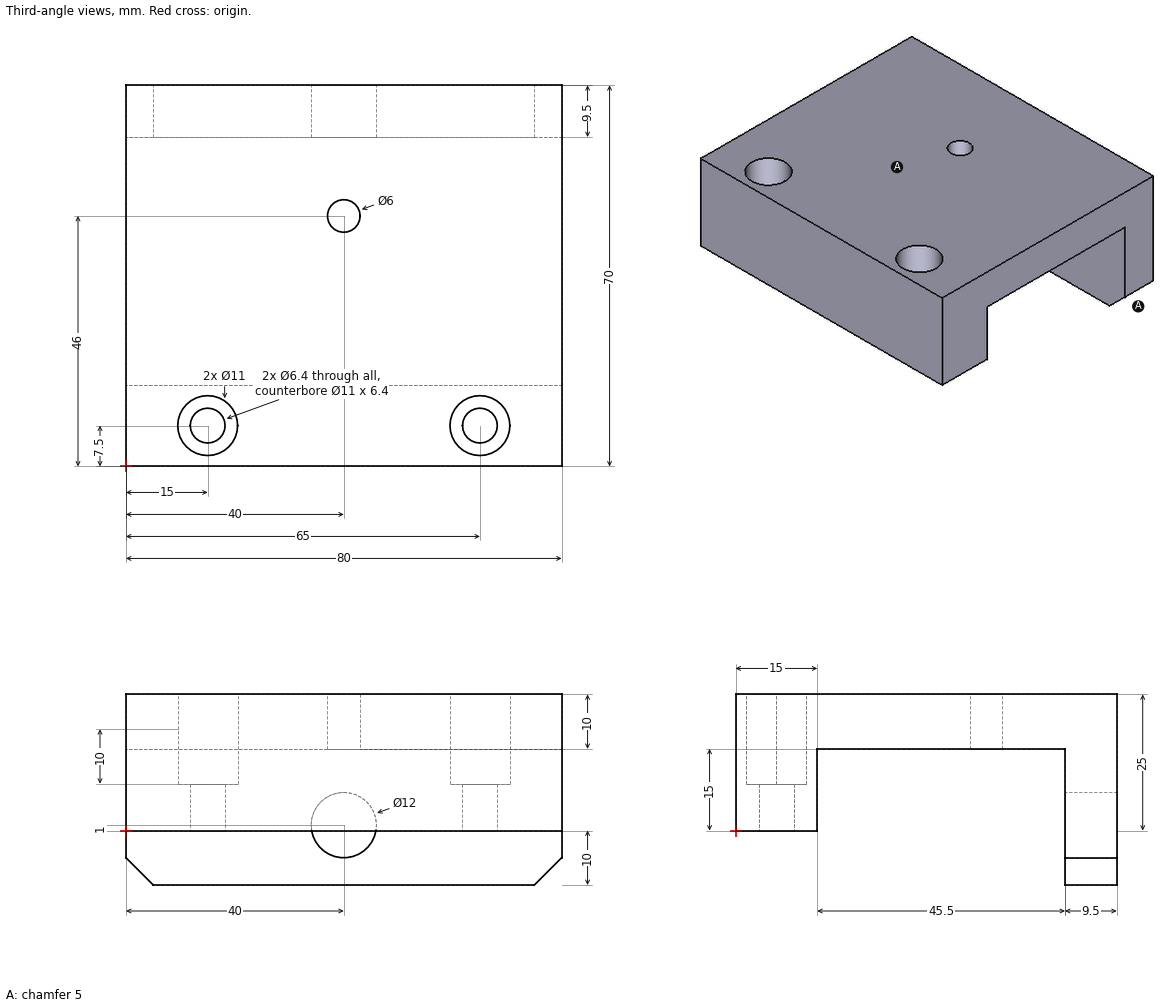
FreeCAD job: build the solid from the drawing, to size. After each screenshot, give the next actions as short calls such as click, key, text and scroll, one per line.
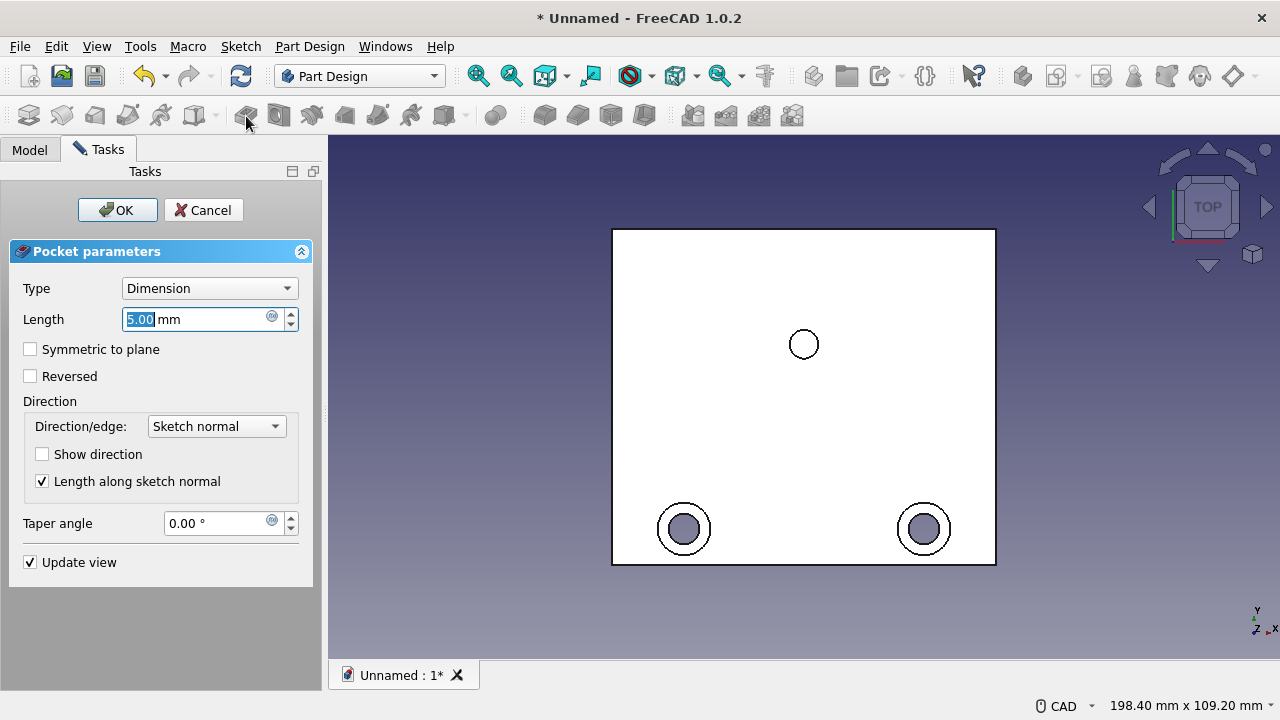
text(10)
key(Tab)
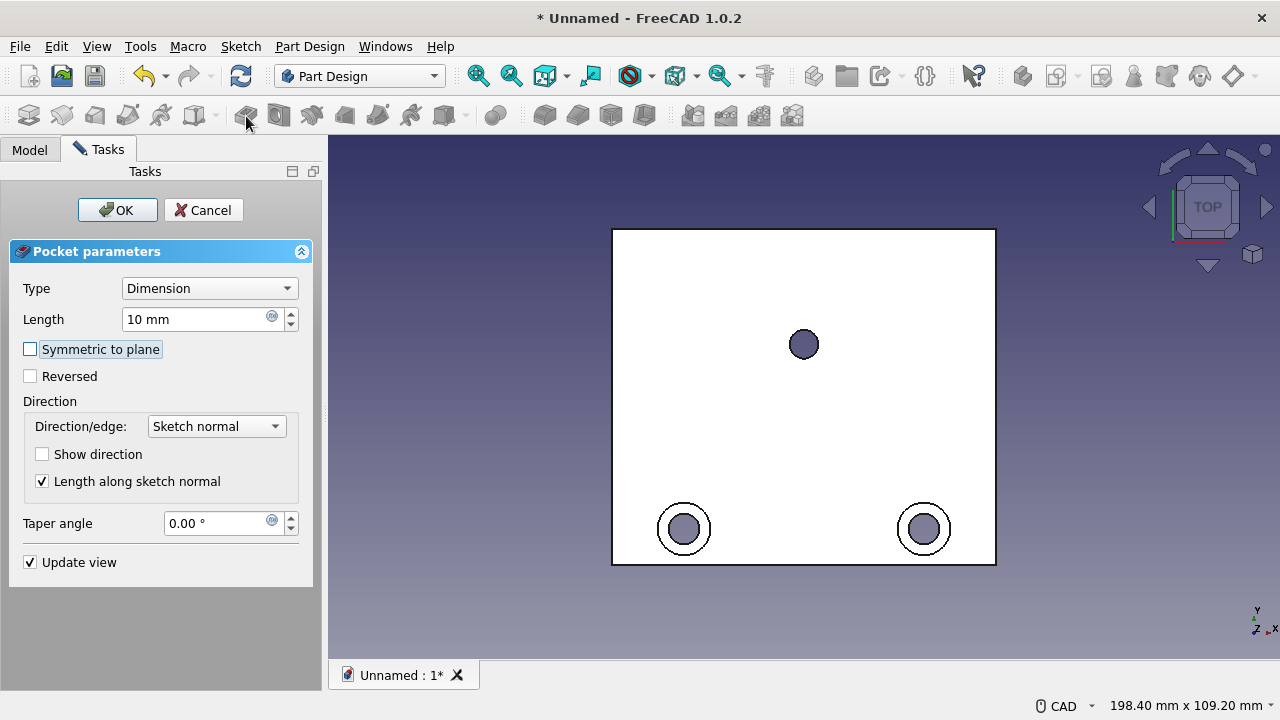
click(118, 210)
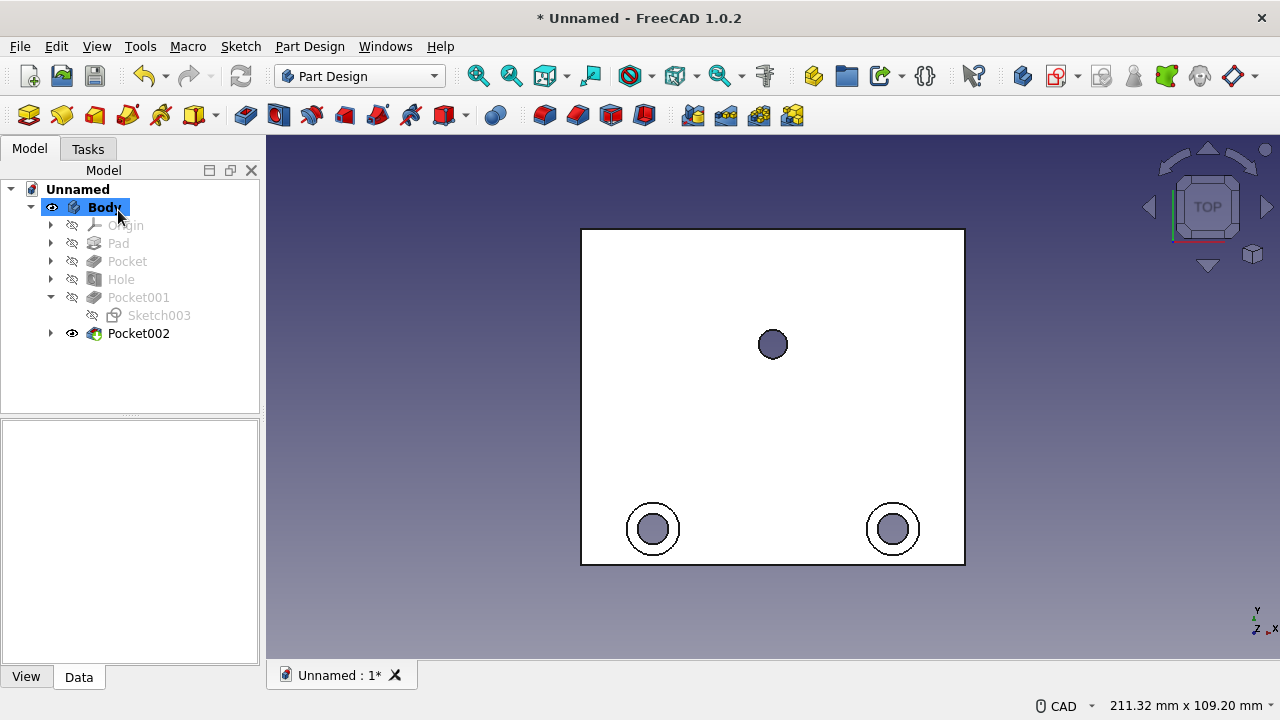
key(5)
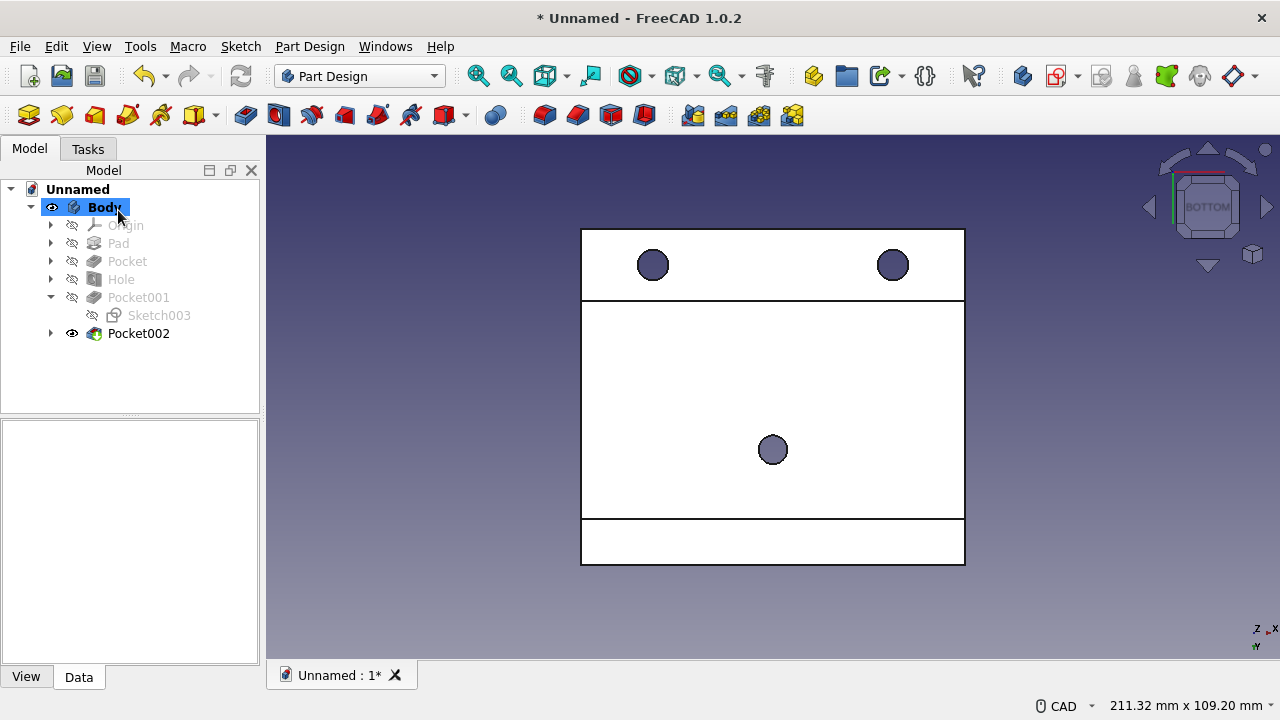
click(828, 264)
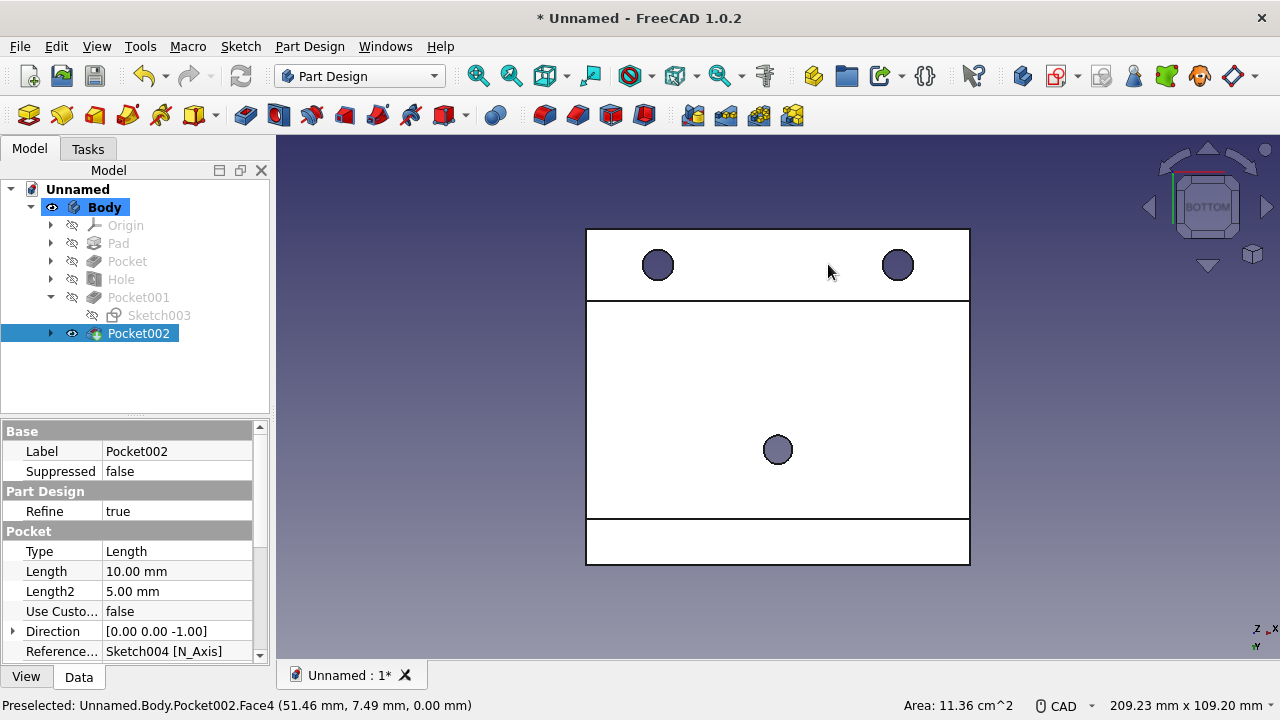
click(1056, 76)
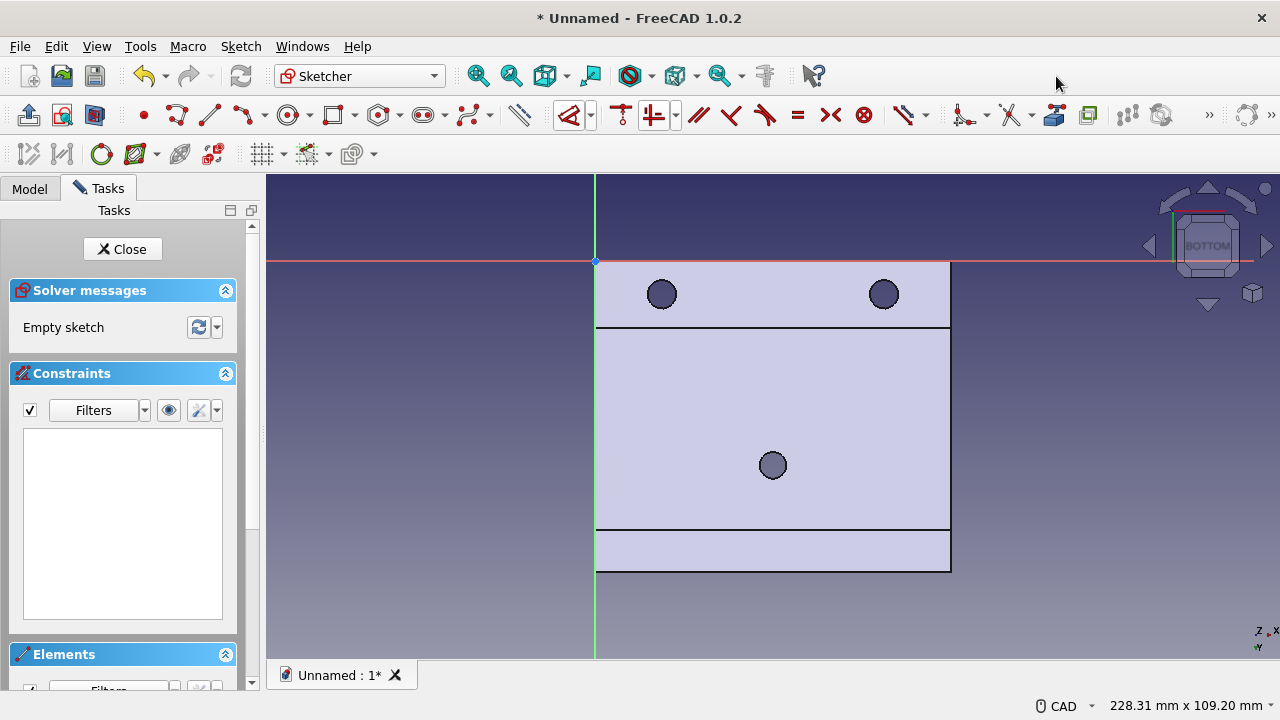
click(332, 116)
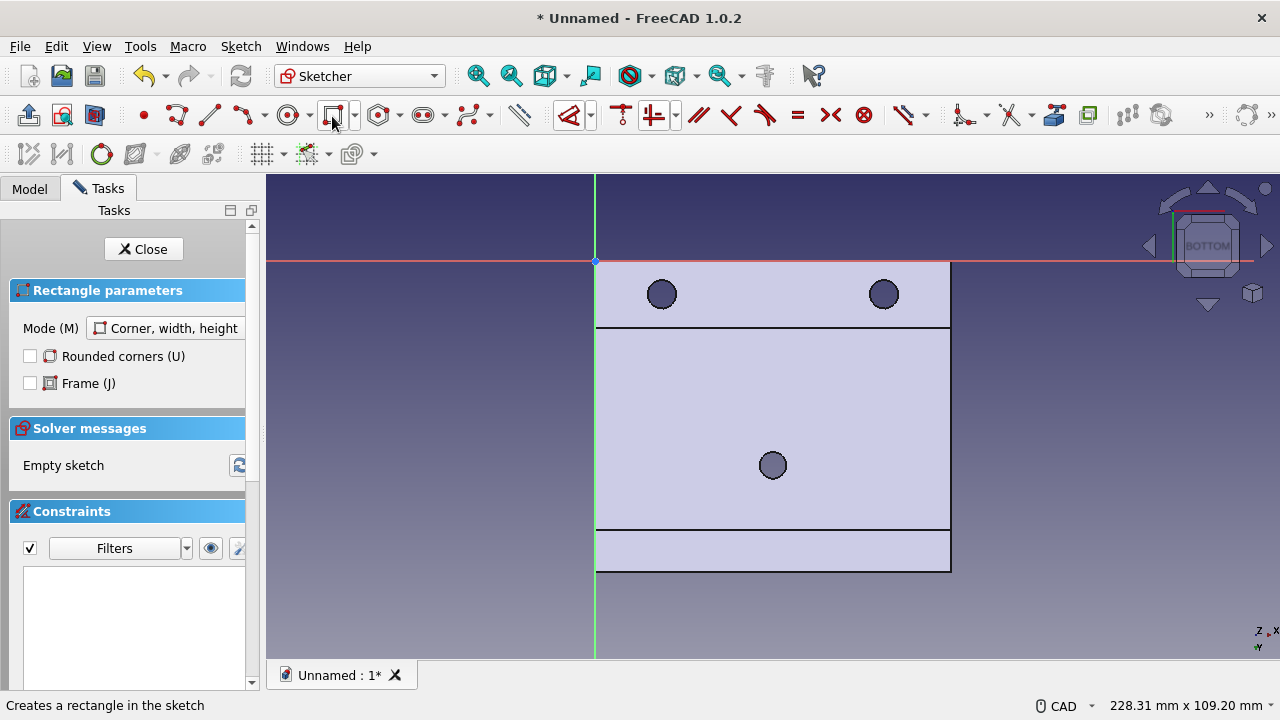
click(595, 530)
move(951, 572)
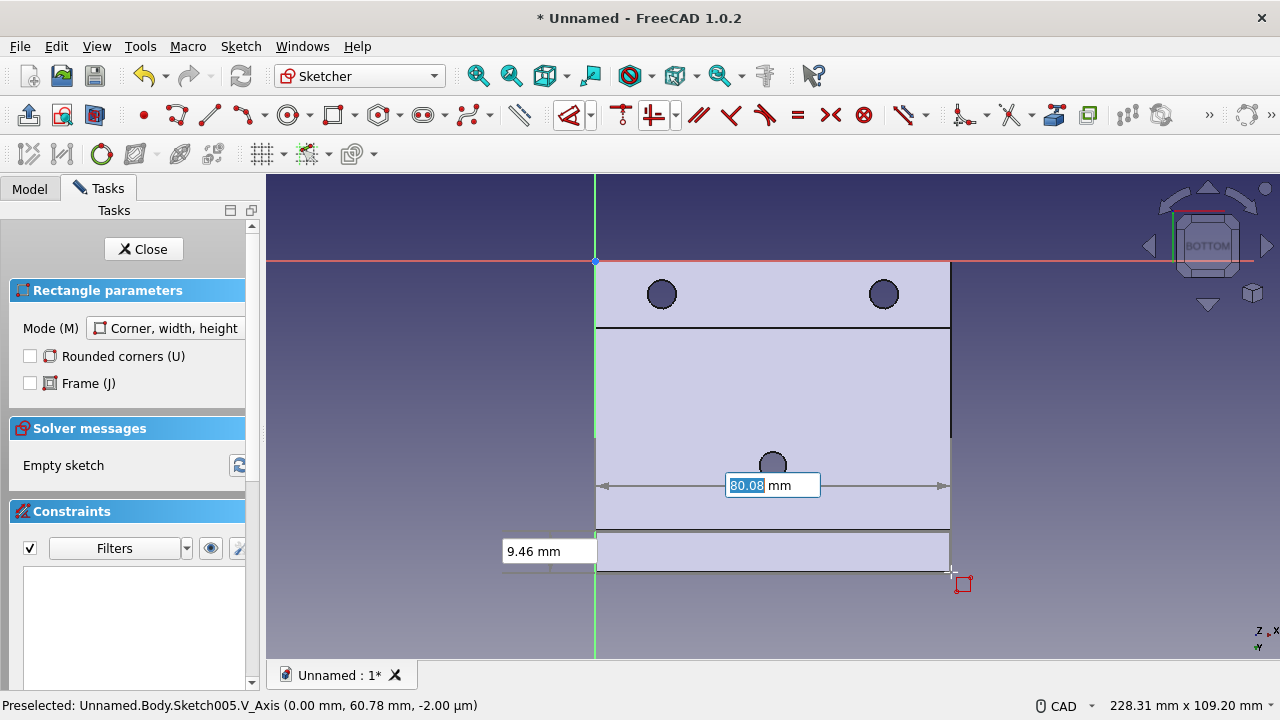
text(80)
key(Tab)
text(9.5)
key(Return)
key(Escape)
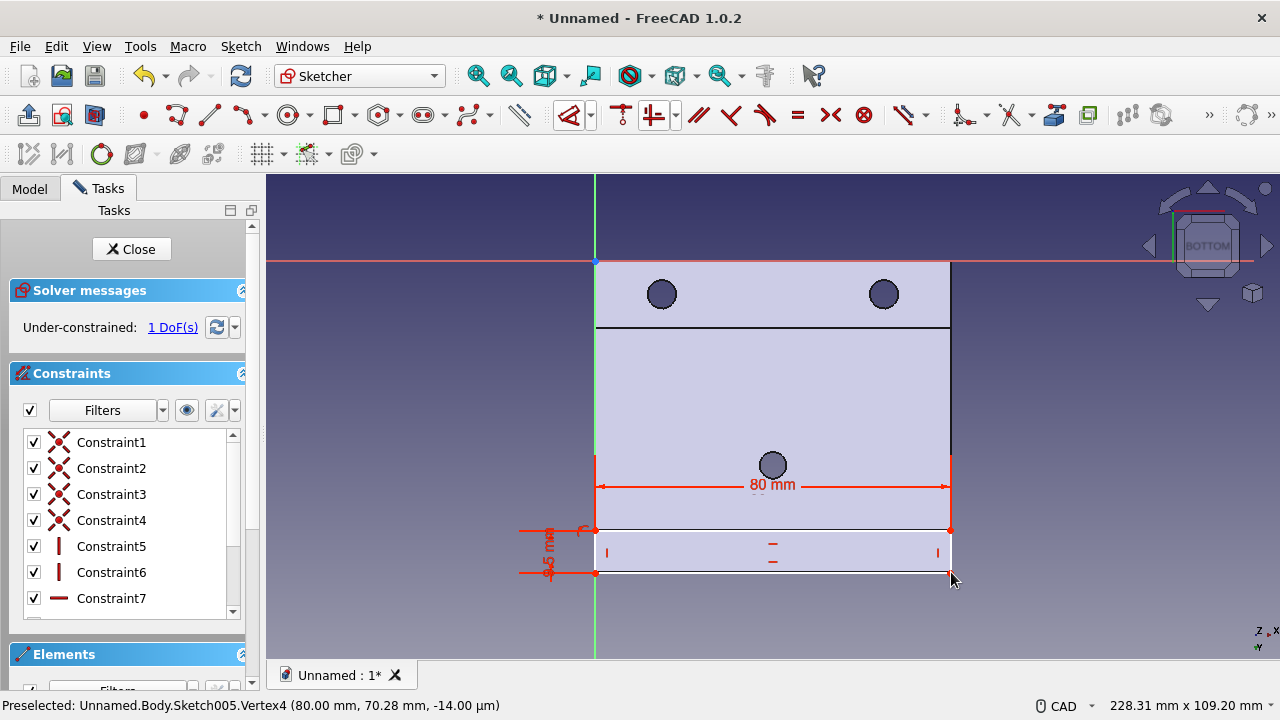
click(595, 573)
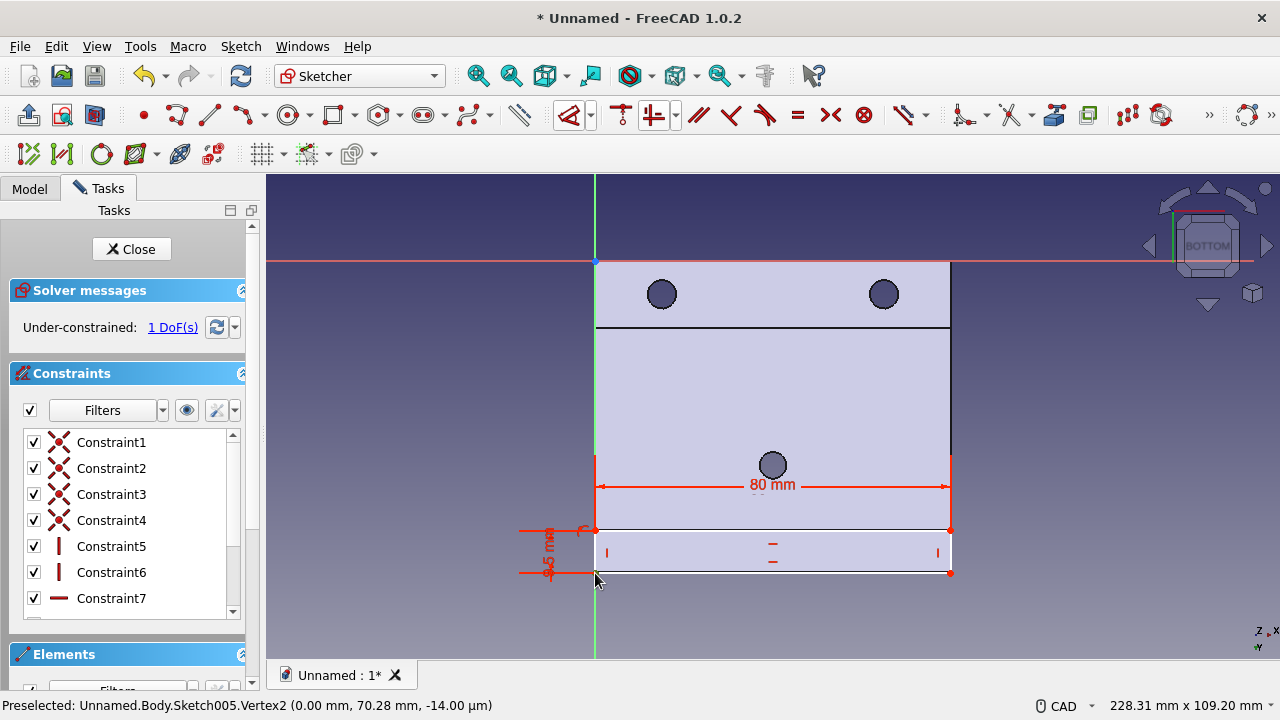
click(590, 116)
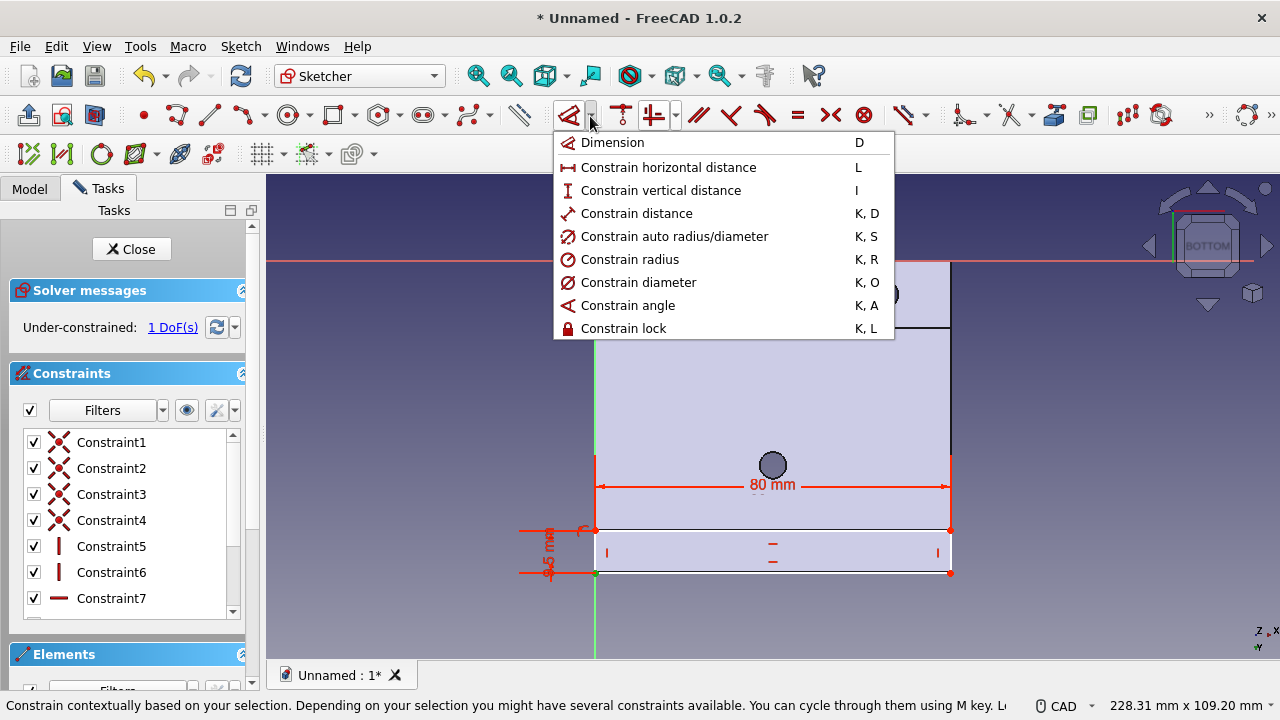
click(724, 190)